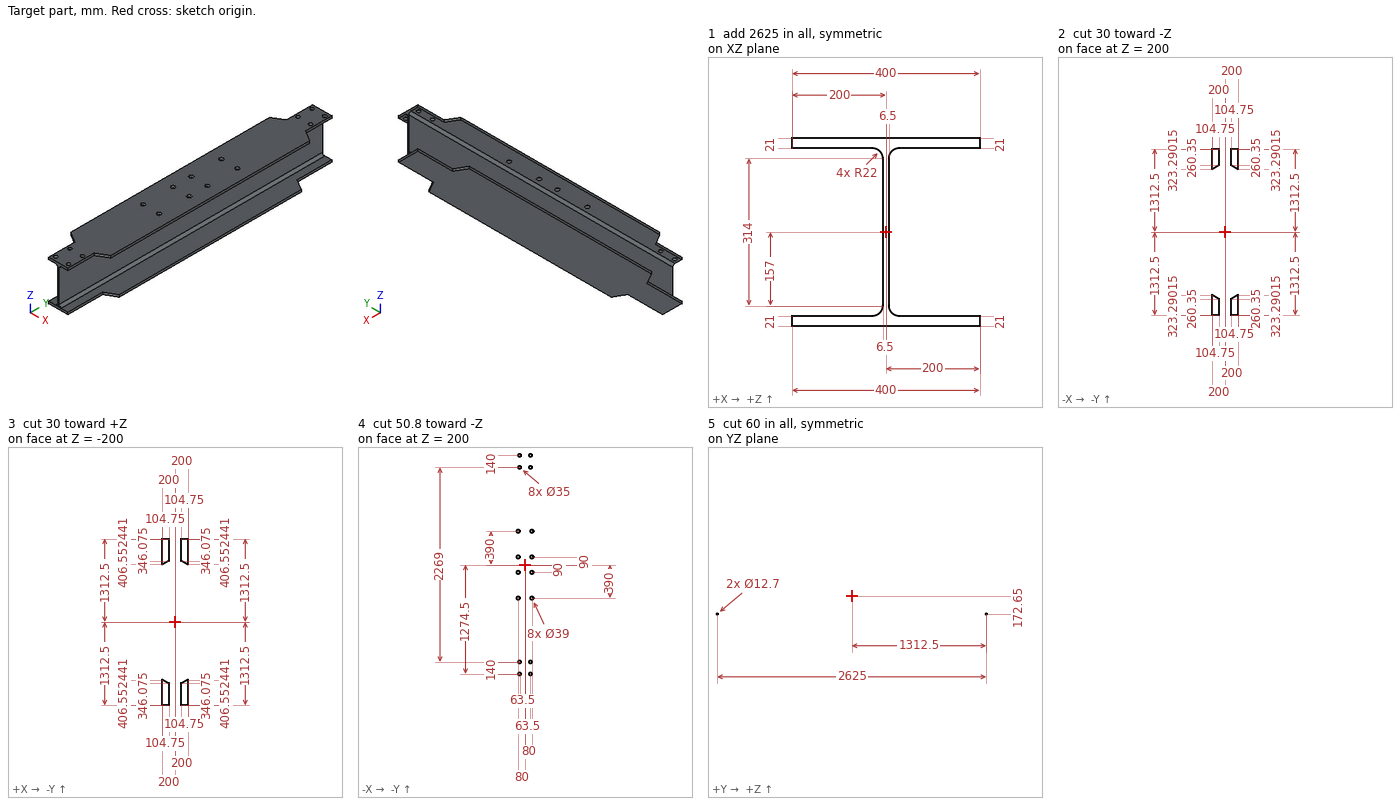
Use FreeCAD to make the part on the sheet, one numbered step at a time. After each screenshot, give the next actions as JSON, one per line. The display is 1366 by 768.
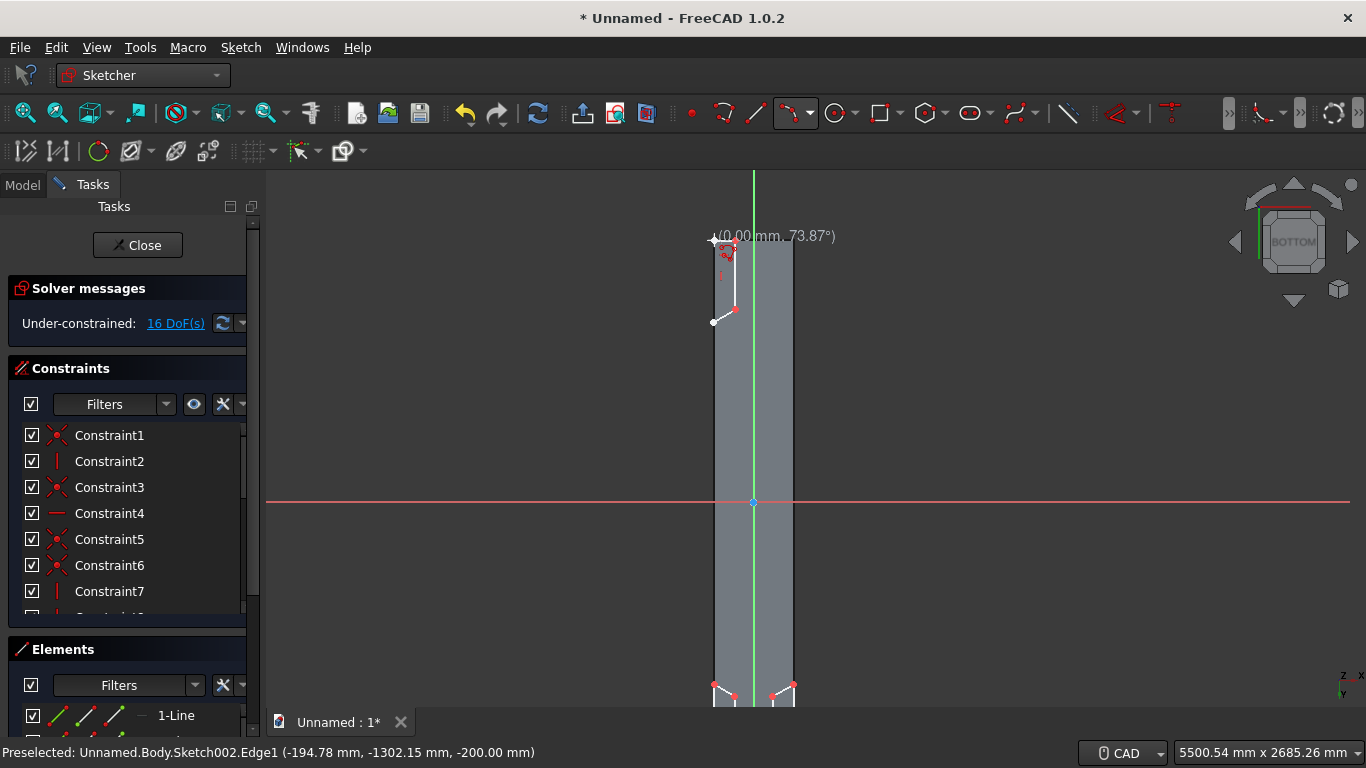
{"action": "scroll", "coordinate": [714, 321], "scroll_direction": "up", "scroll_amount": 2}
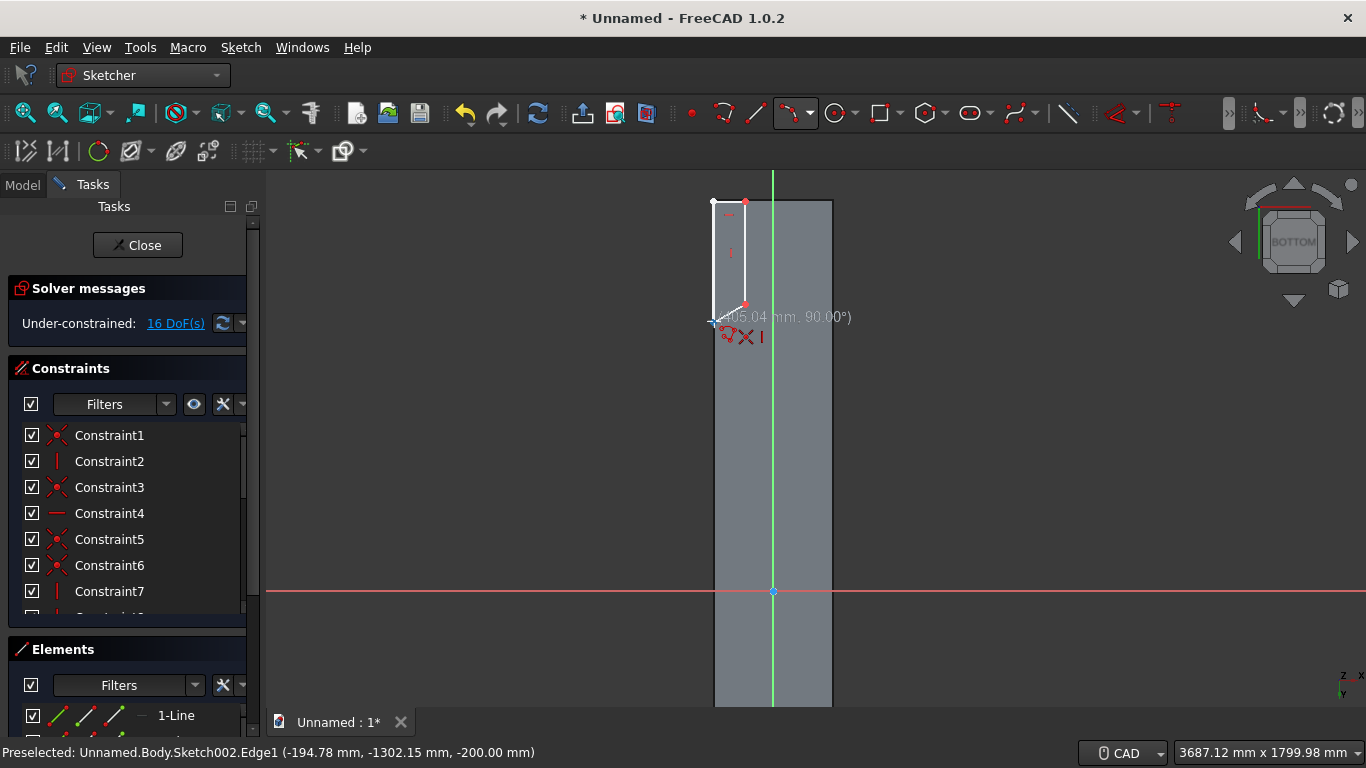
{"action": "left_click", "coordinate": [714, 323]}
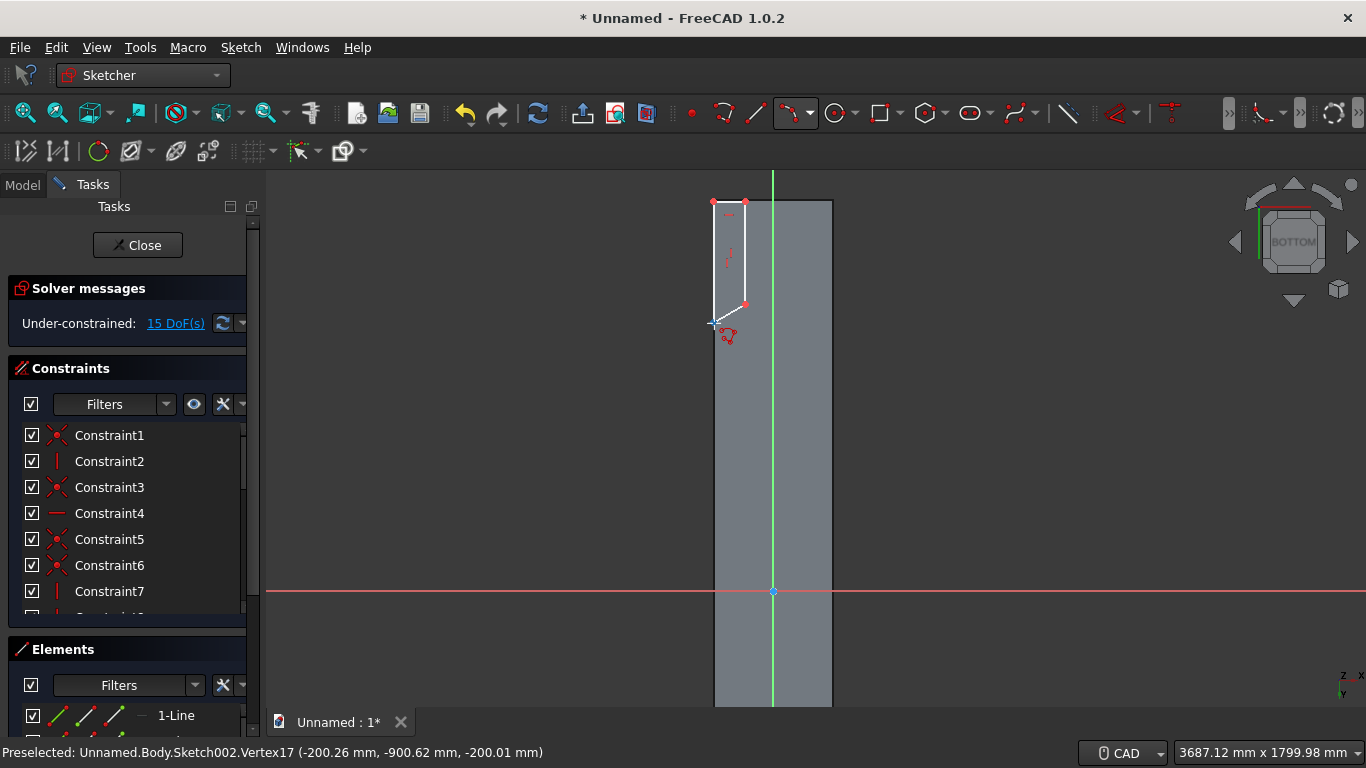
{"action": "left_click", "coordinate": [833, 321]}
{"action": "left_click", "coordinate": [833, 200]}
{"action": "left_click", "coordinate": [802, 200]}
{"action": "left_click", "coordinate": [802, 303]}
{"action": "left_click", "coordinate": [833, 322]}
{"action": "key", "text": "Escape"}
{"action": "key", "text": "Escape"}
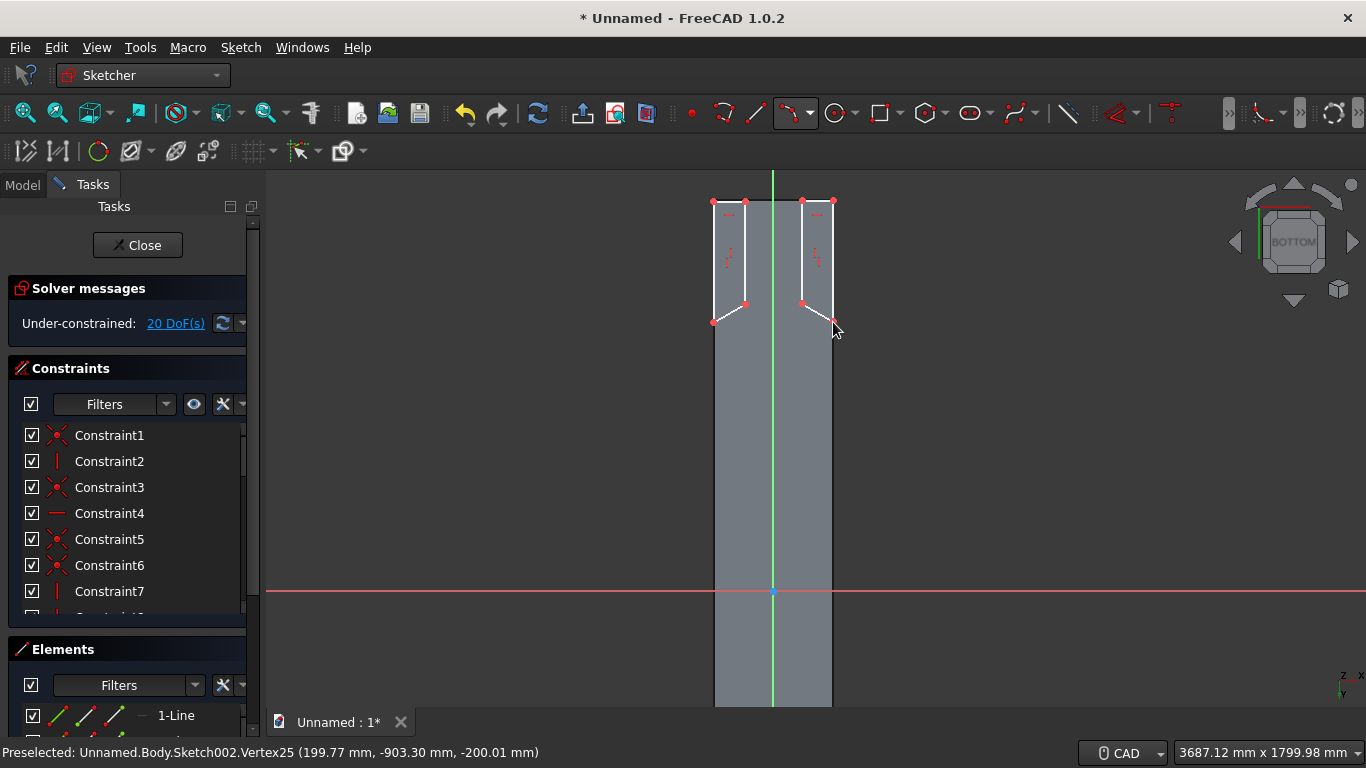
{"action": "left_click", "coordinate": [1116, 114]}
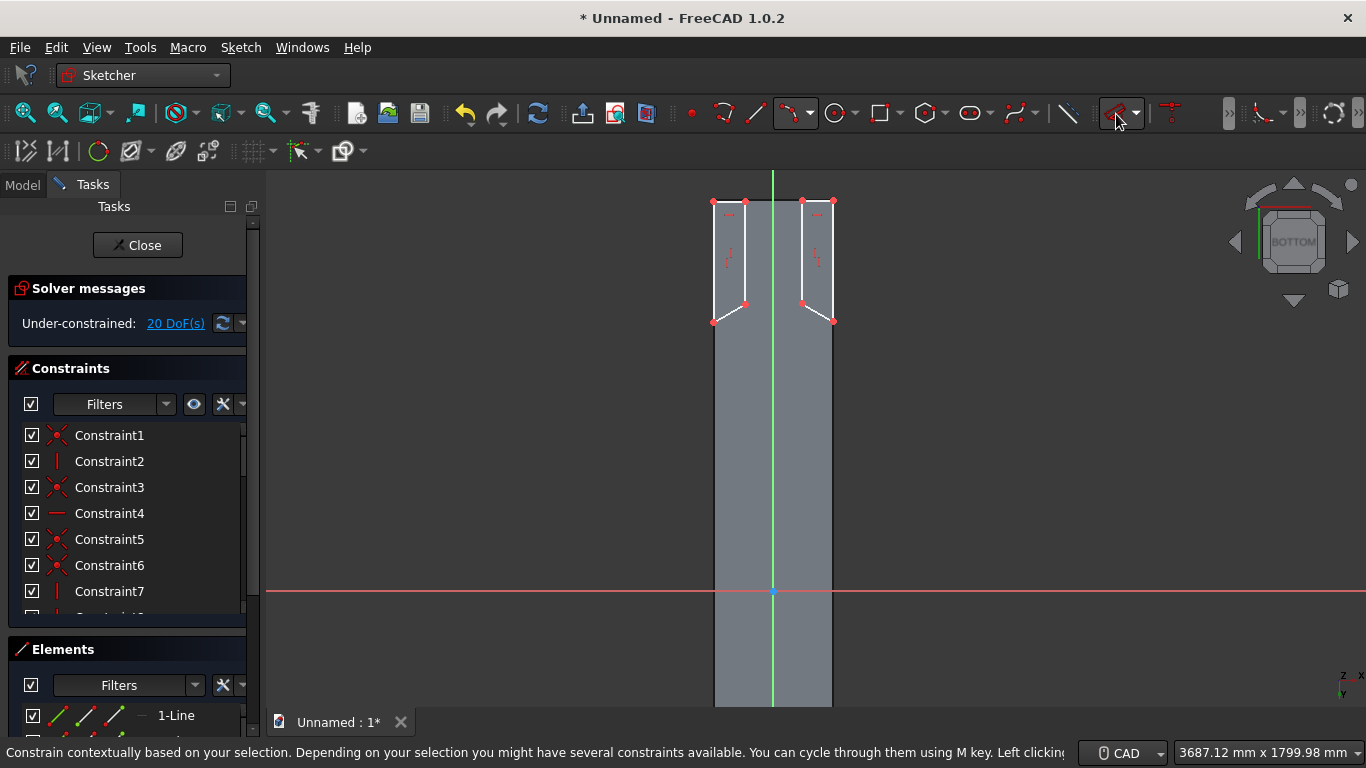
{"action": "scroll", "coordinate": [726, 314], "scroll_direction": "down", "scroll_amount": 4}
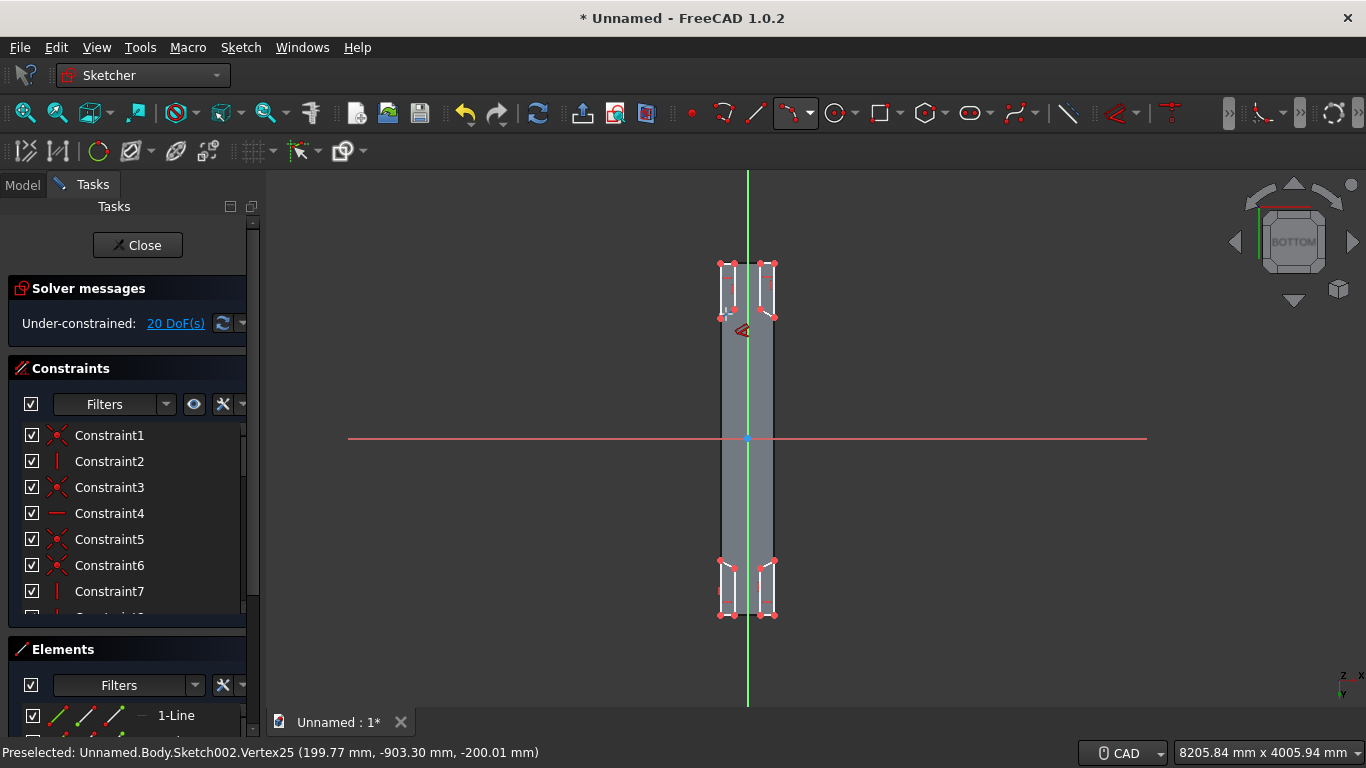
{"action": "scroll", "coordinate": [774, 561], "scroll_direction": "up", "scroll_amount": 2}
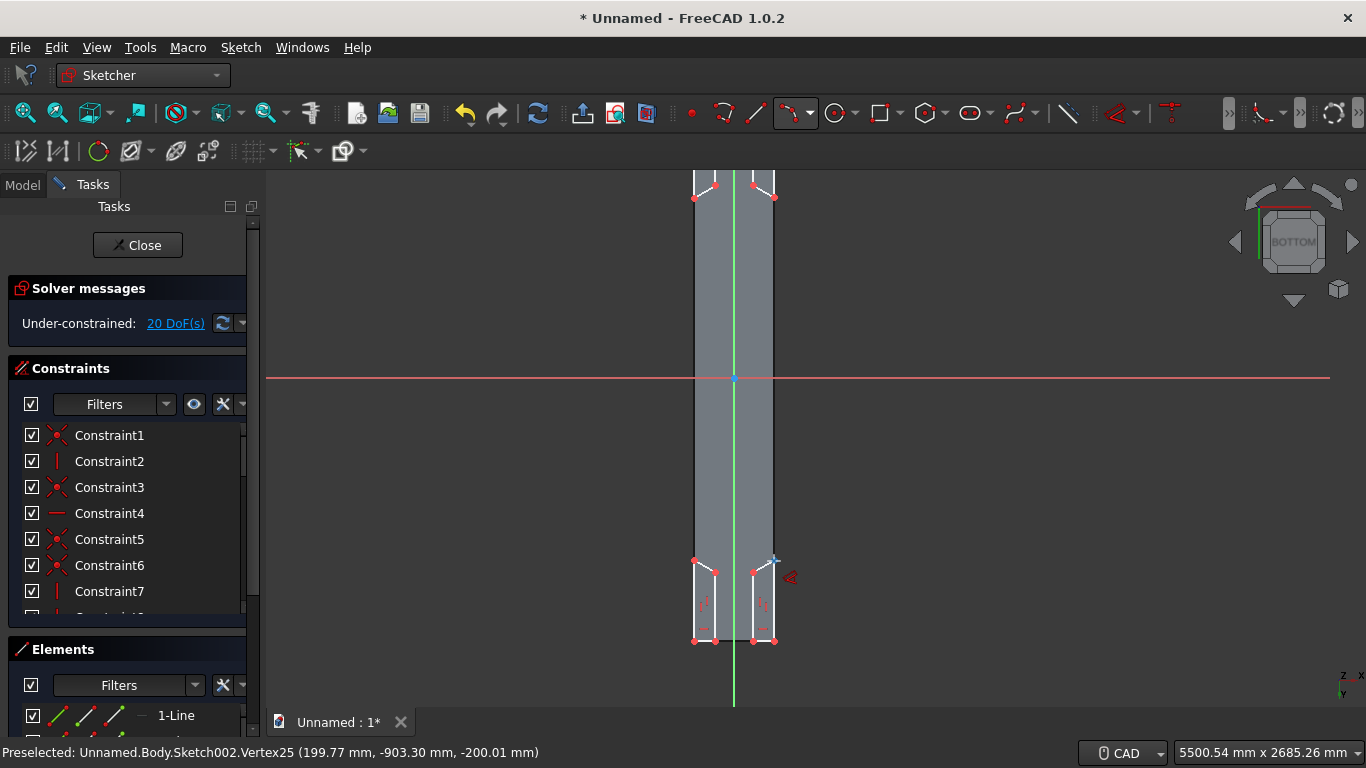
{"action": "left_click", "coordinate": [774, 561]}
{"action": "left_click", "coordinate": [754, 344]}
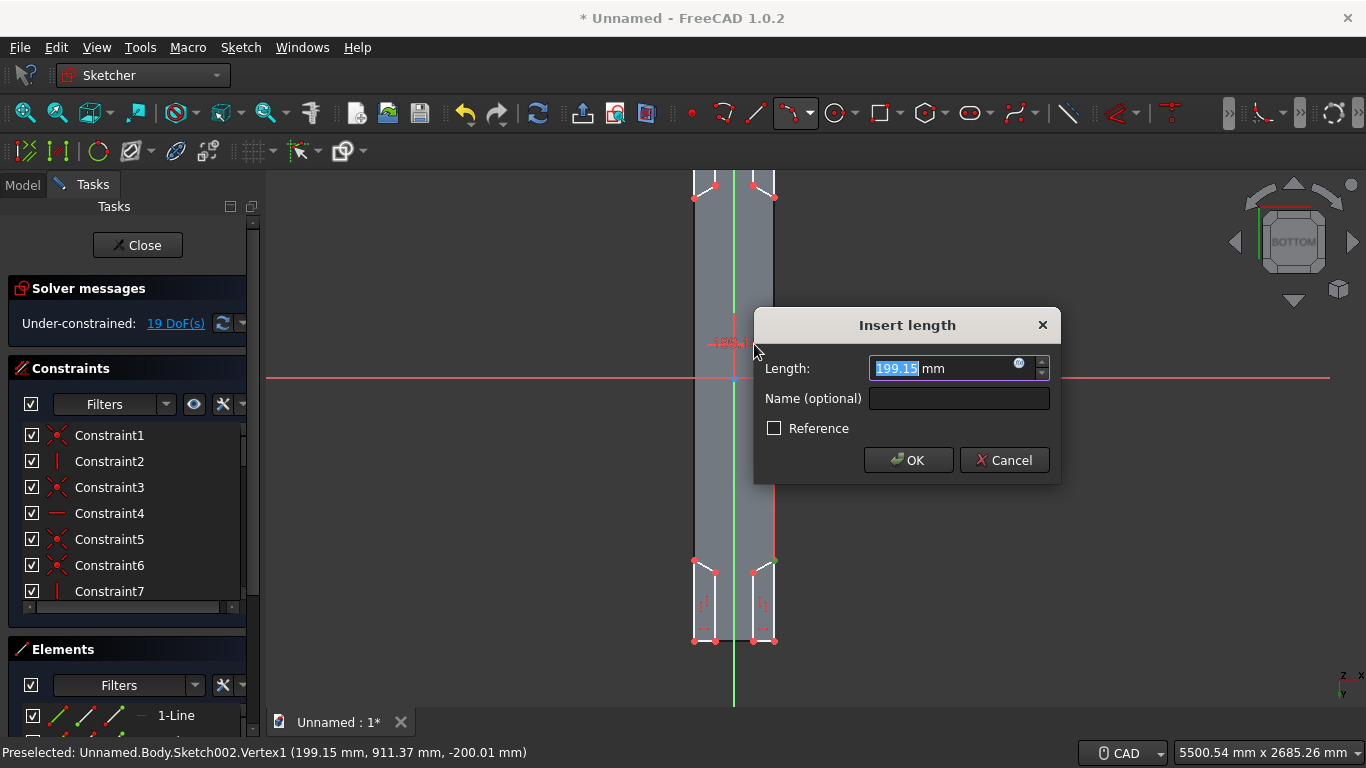
{"action": "type", "text": "200"}
{"action": "key", "text": "Return"}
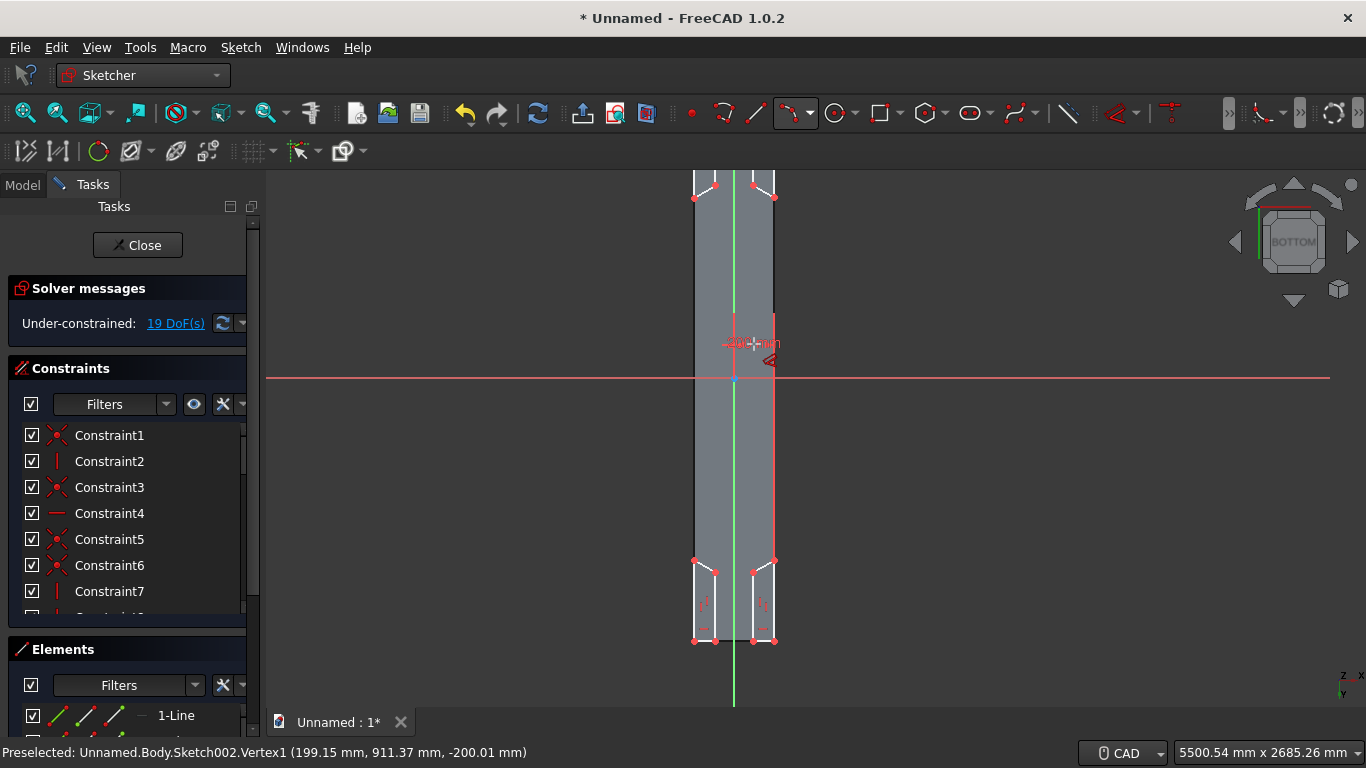
{"action": "left_click", "coordinate": [694, 560]}
{"action": "left_click", "coordinate": [714, 320]}